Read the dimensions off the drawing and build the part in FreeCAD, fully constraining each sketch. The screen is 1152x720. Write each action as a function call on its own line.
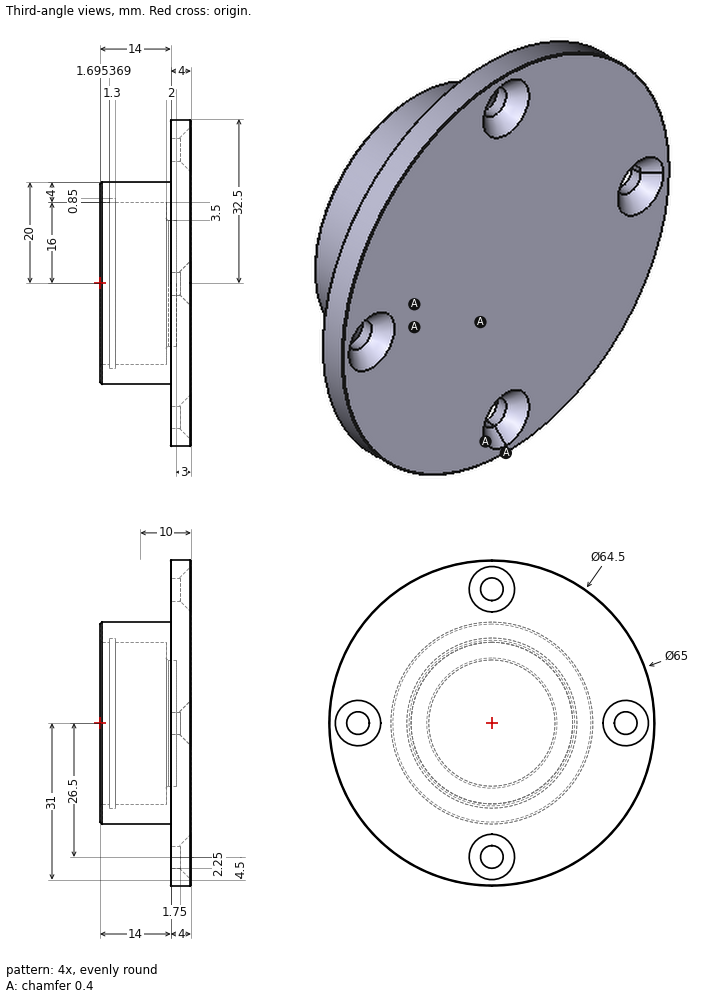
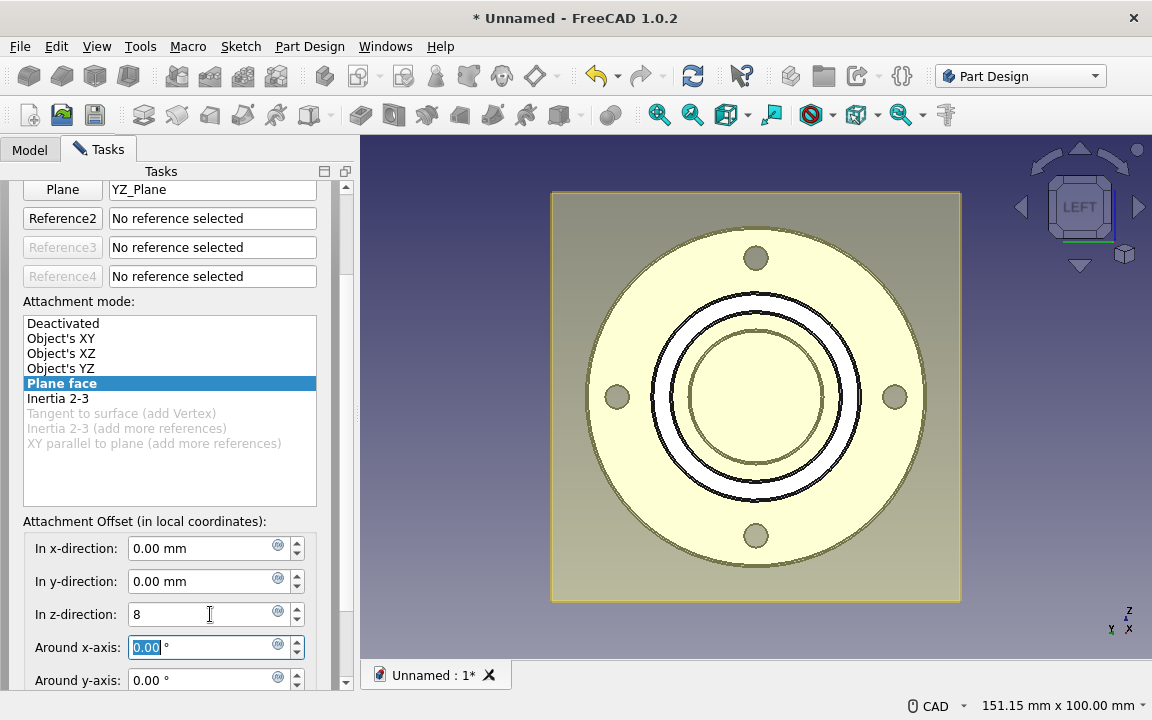
scroll(346, 436, up, 3)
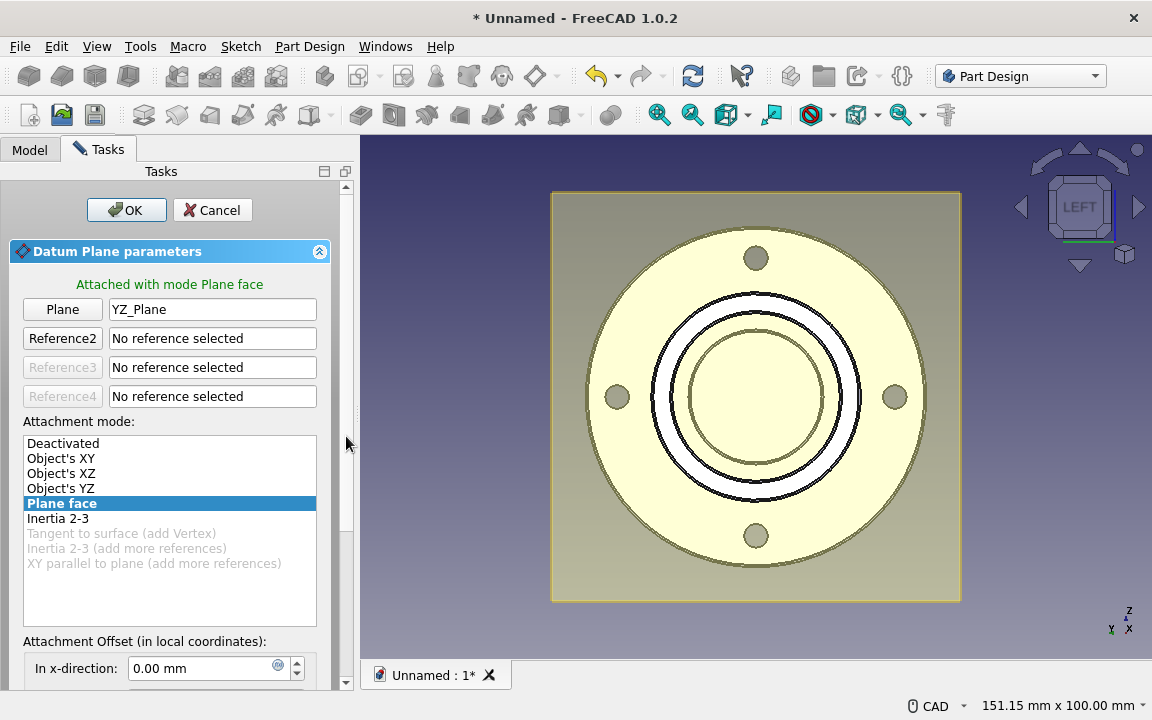
click(127, 210)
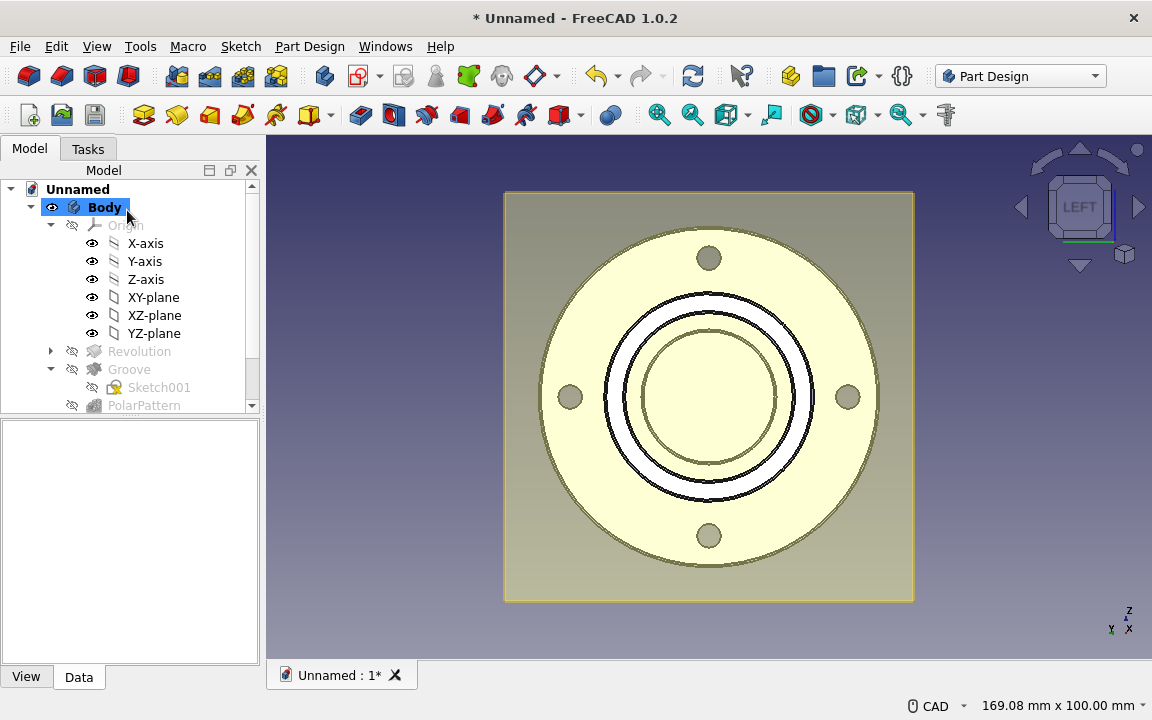
scroll(101, 293, down, 3)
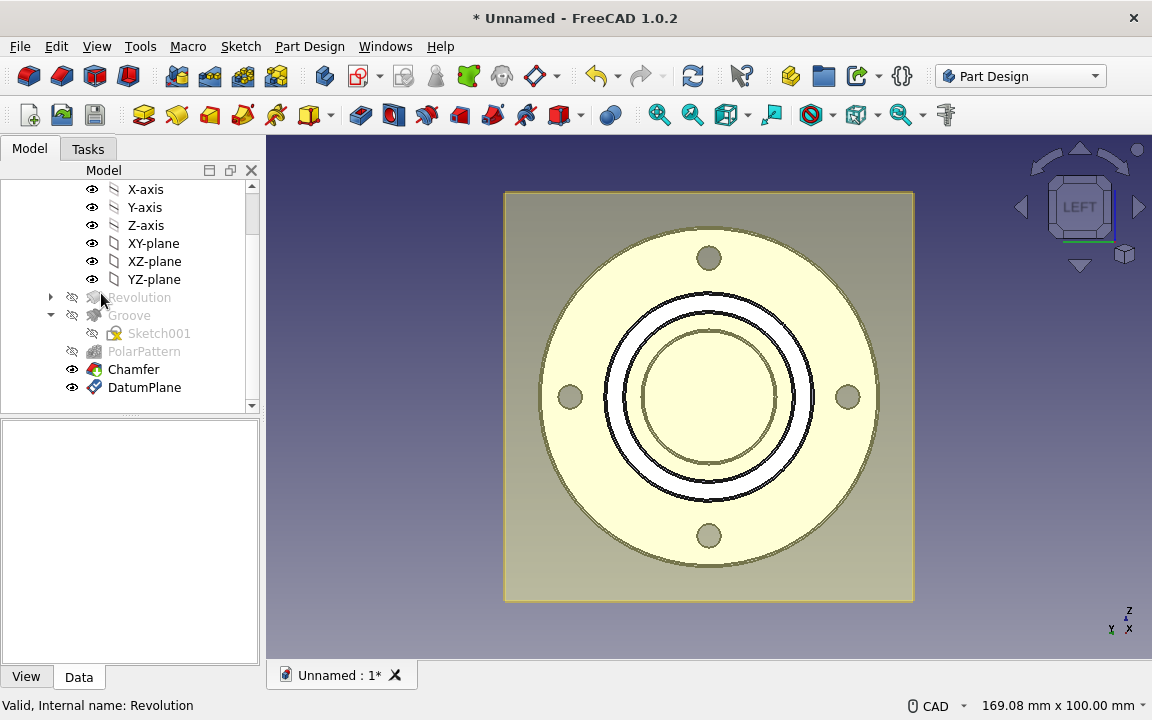
click(117, 387)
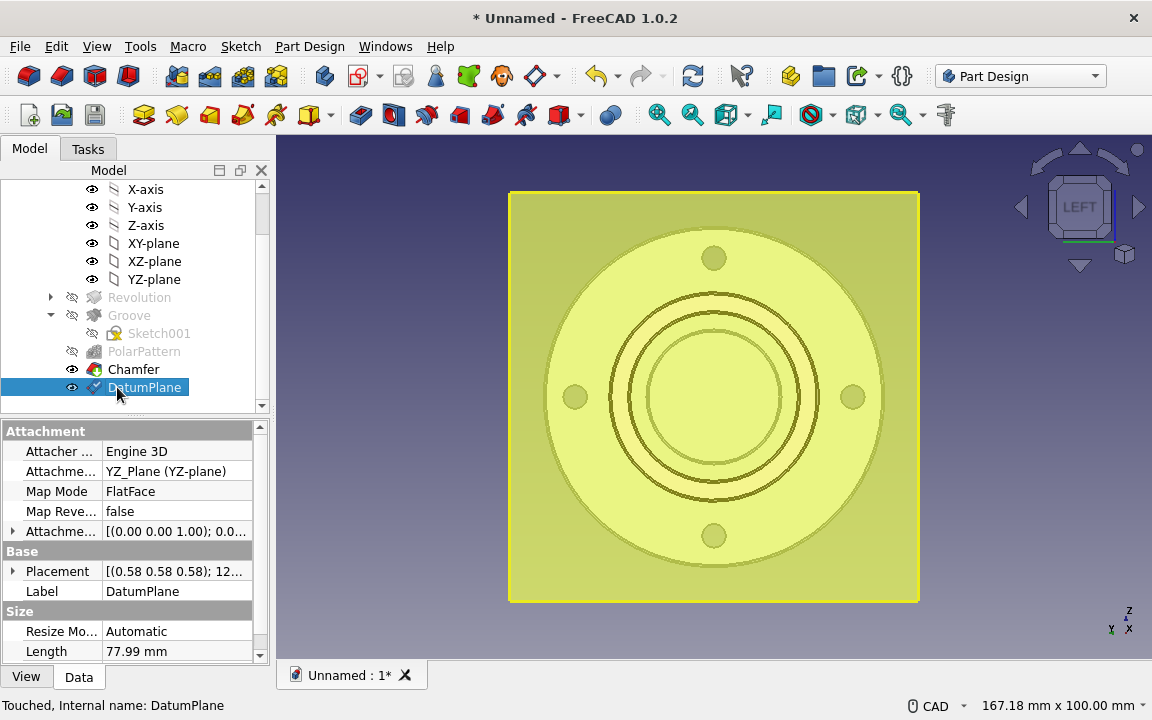
click(358, 76)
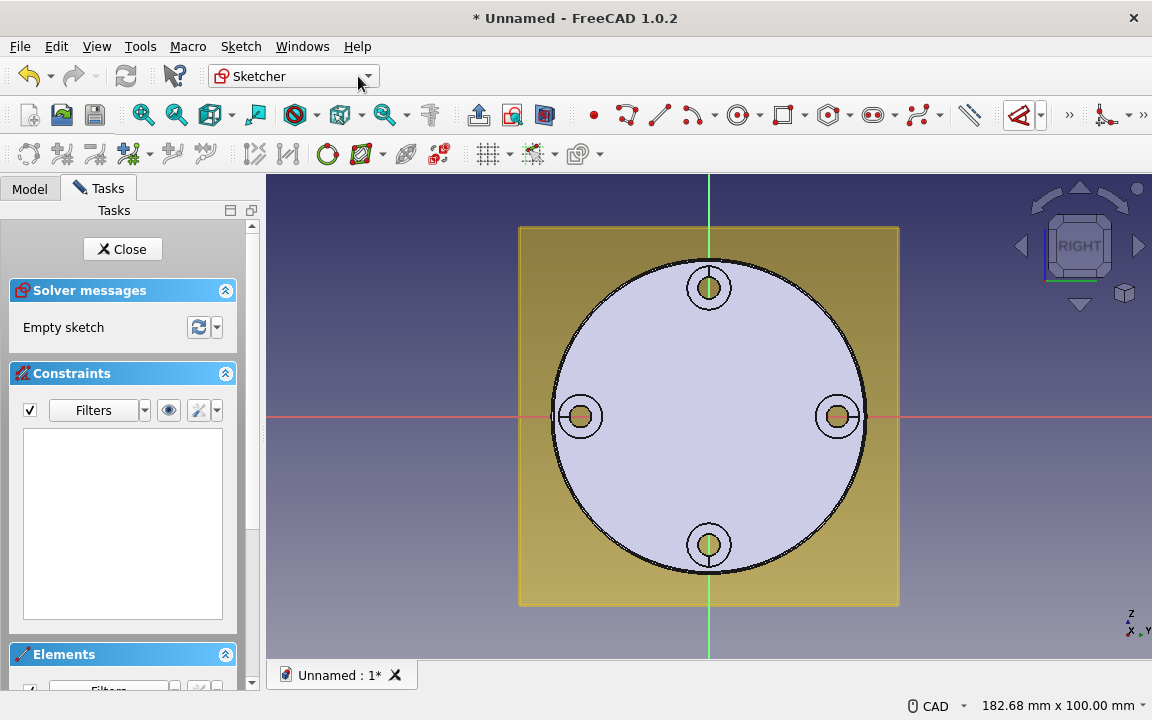
key(q)
key(s)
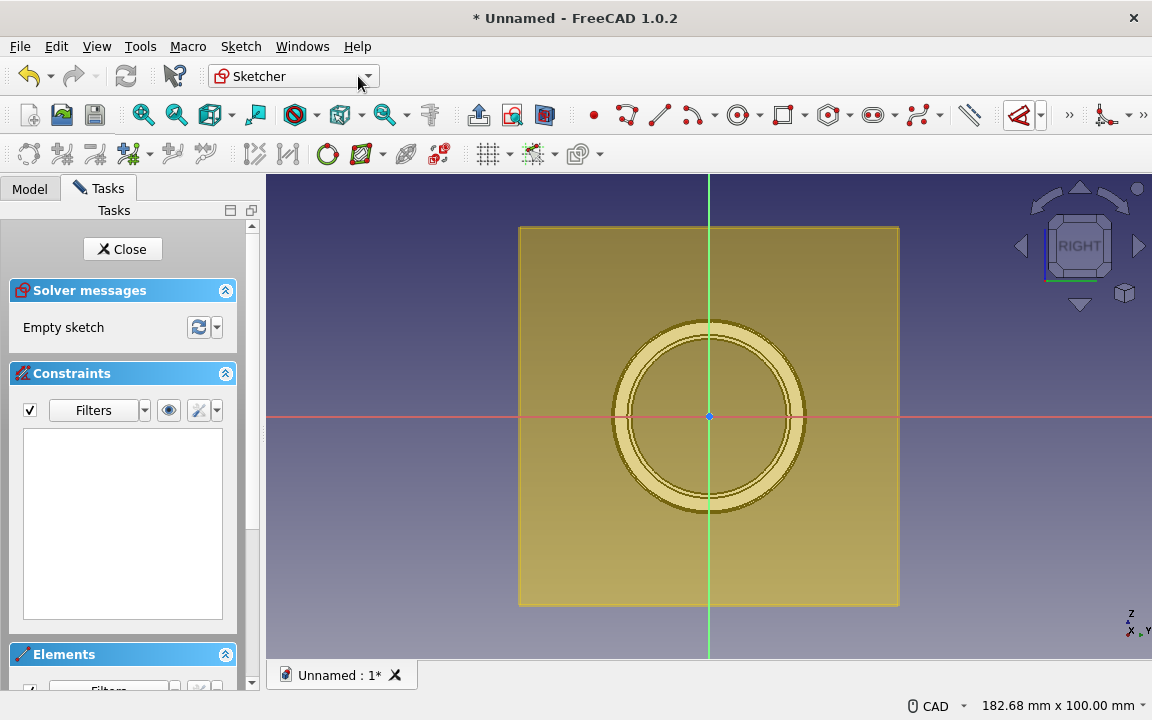
click(738, 116)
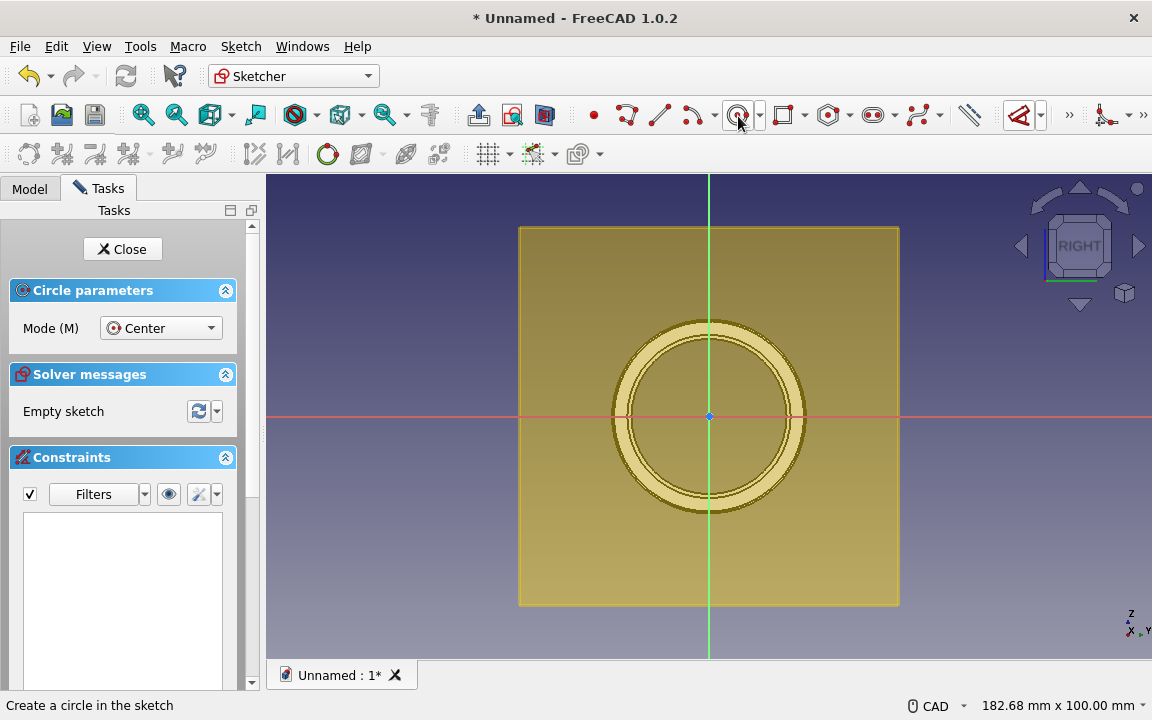
click(709, 416)
move(820, 305)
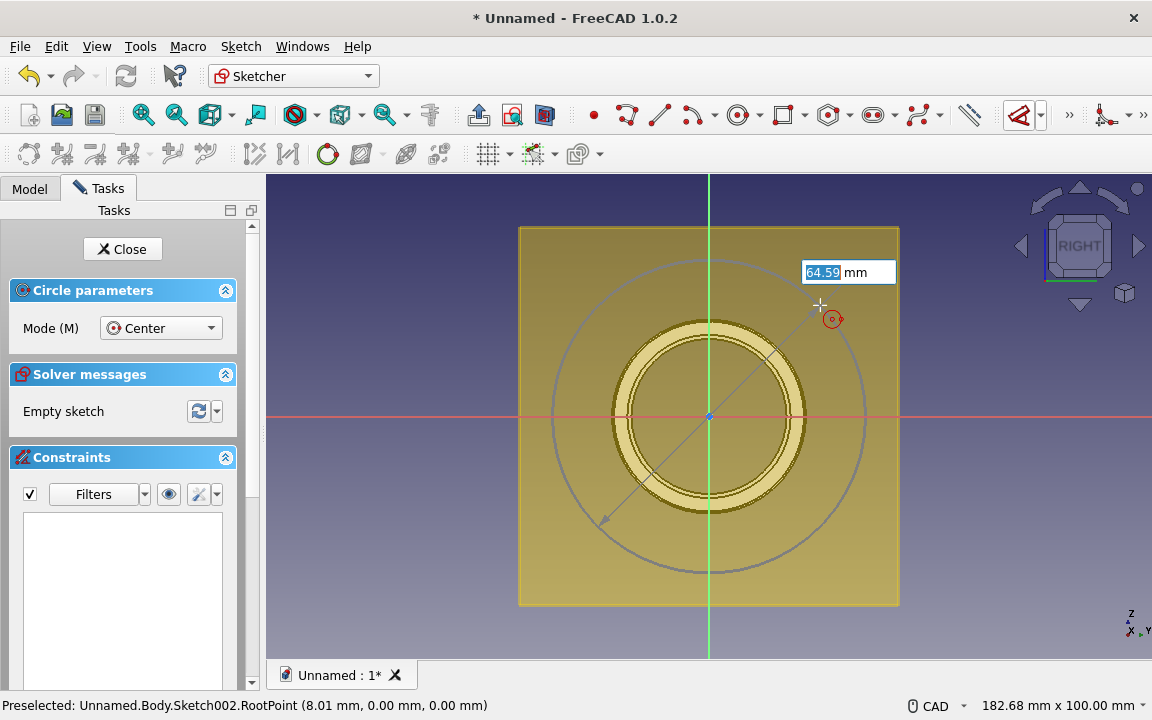
text(65)
key(Return)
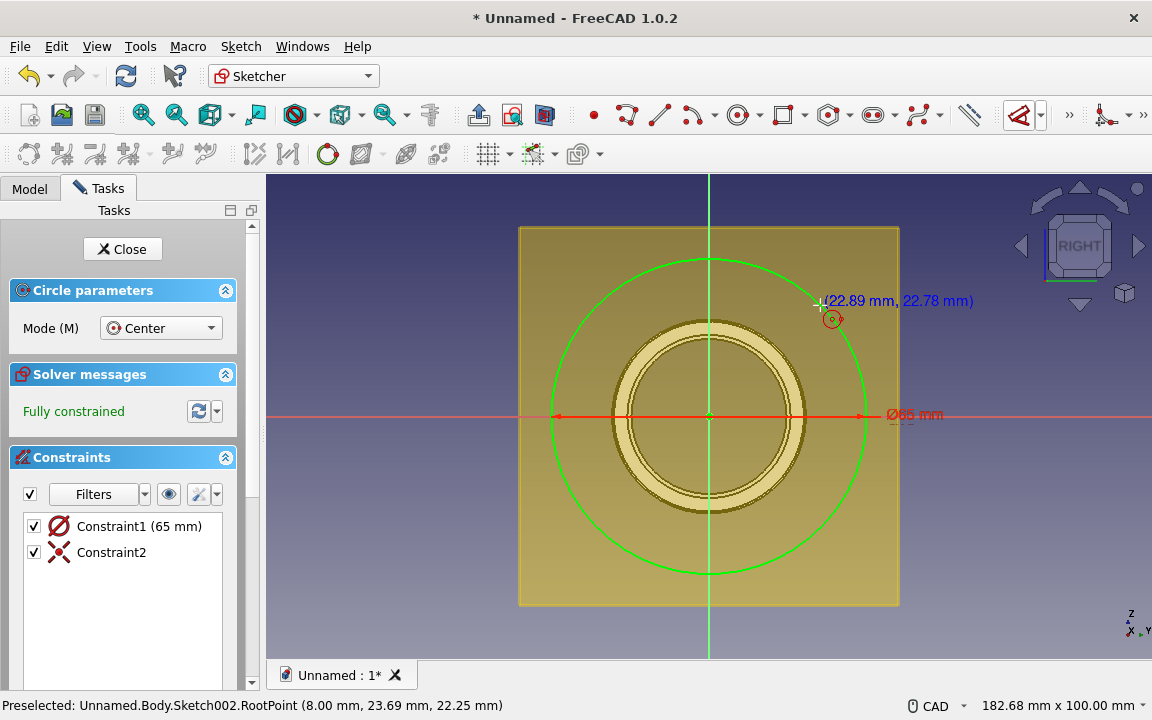
click(709, 416)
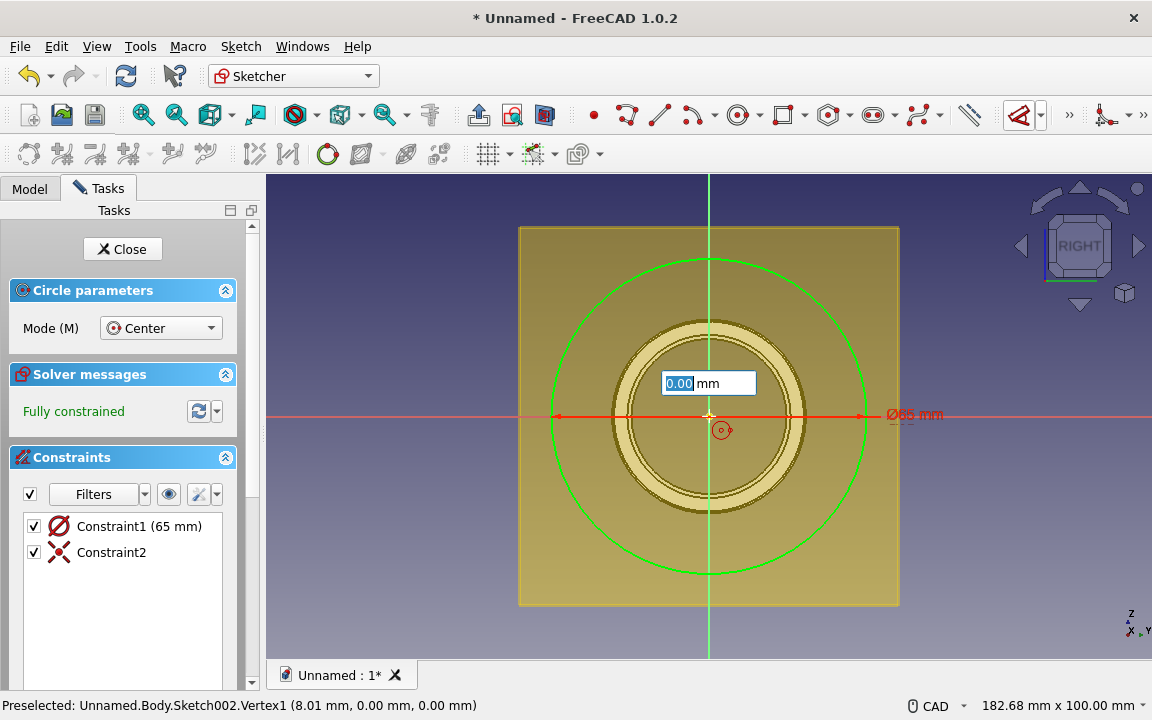
scroll(820, 306, up, 13)
move(807, 301)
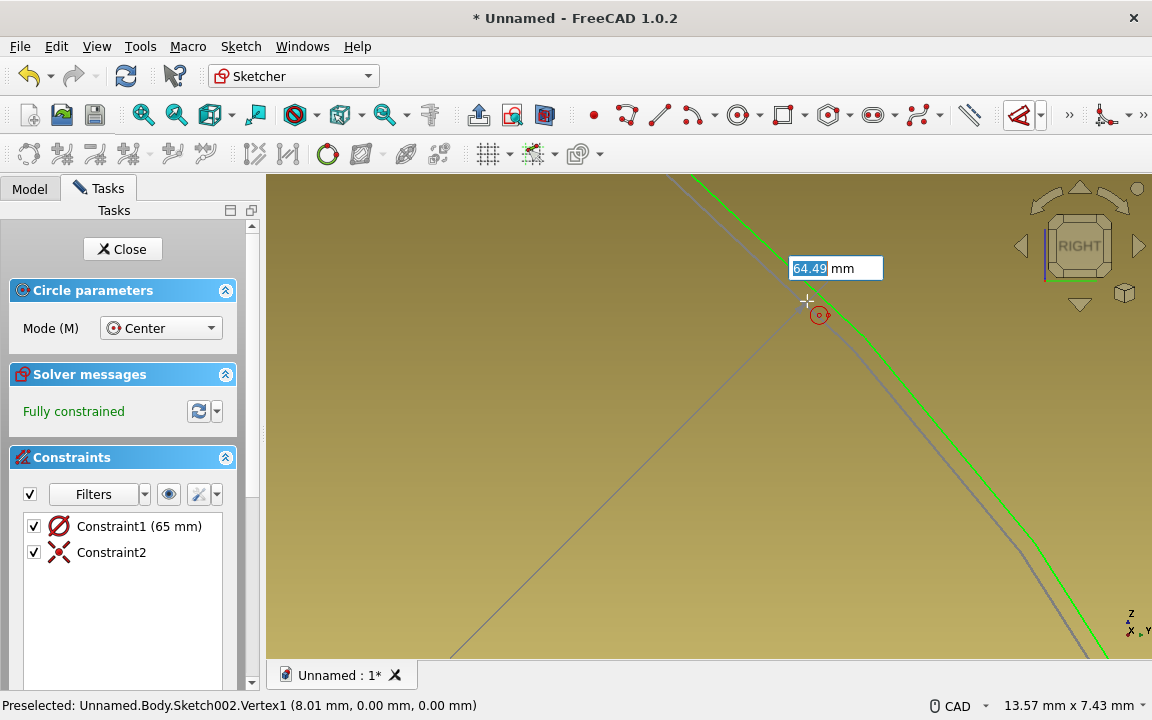
text(64.5)
key(Return)
key(Escape)